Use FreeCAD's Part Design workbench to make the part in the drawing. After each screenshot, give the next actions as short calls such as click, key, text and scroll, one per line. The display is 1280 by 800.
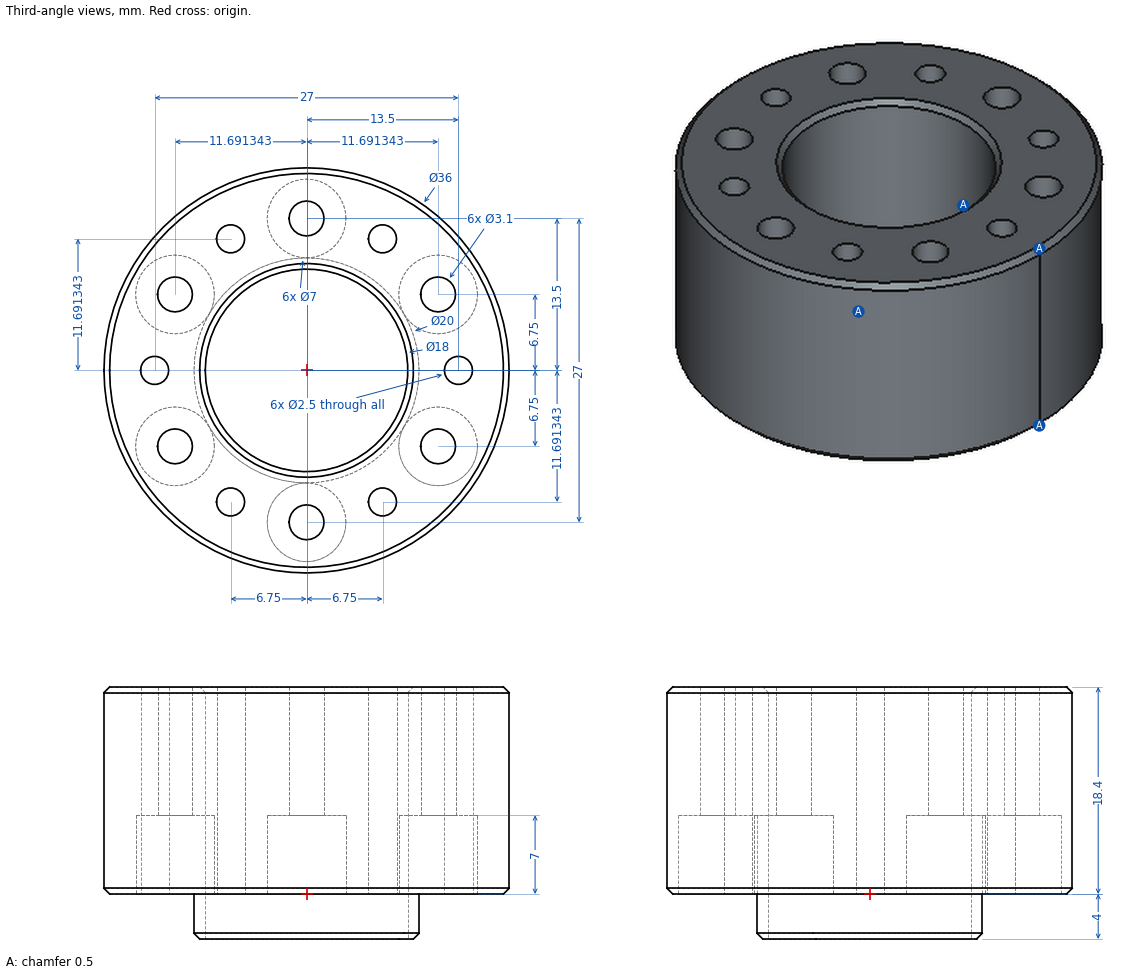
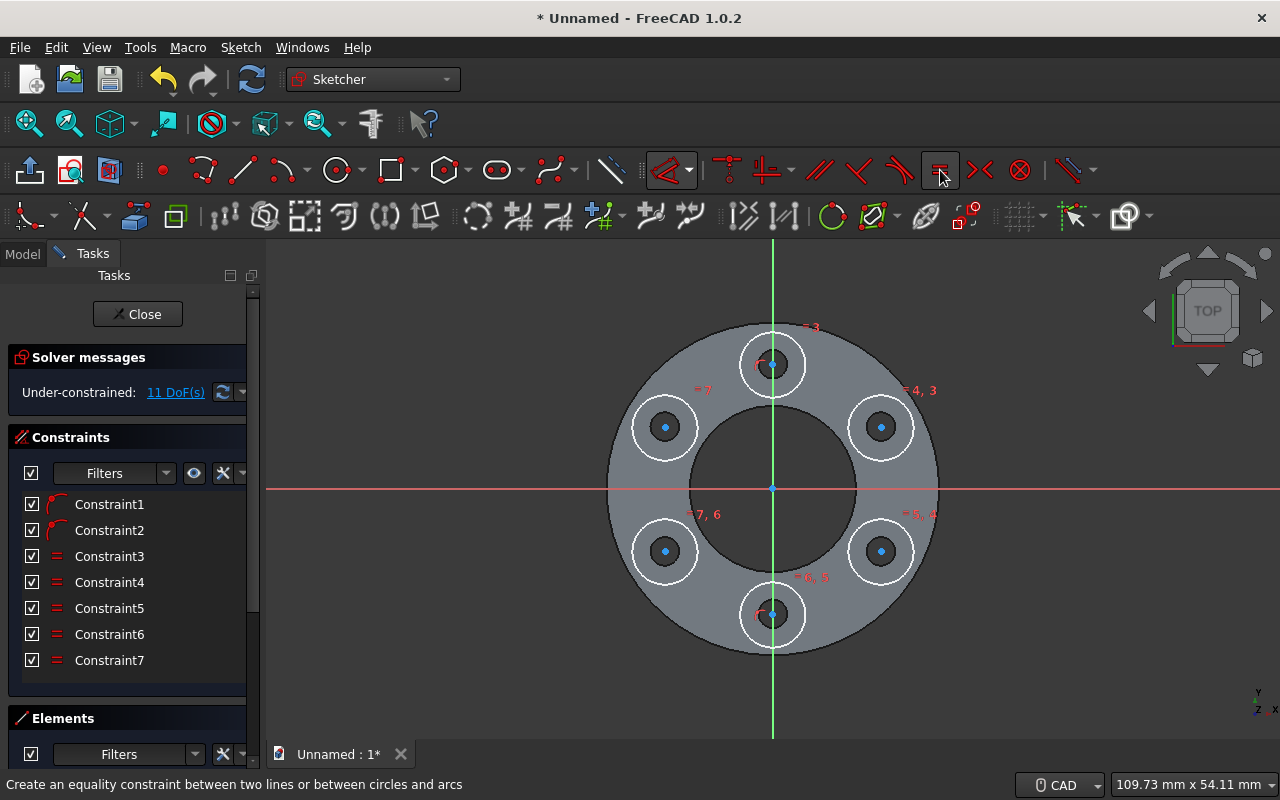
click(796, 342)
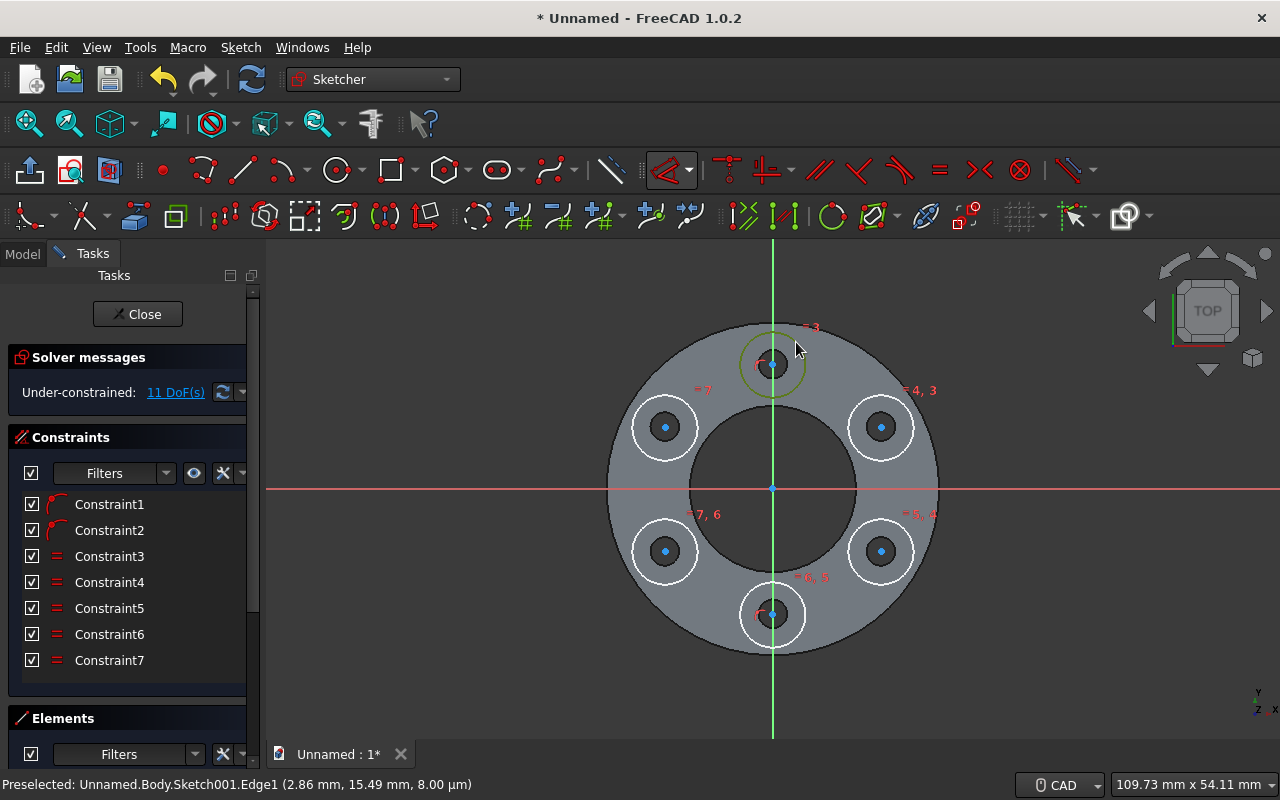
click(692, 170)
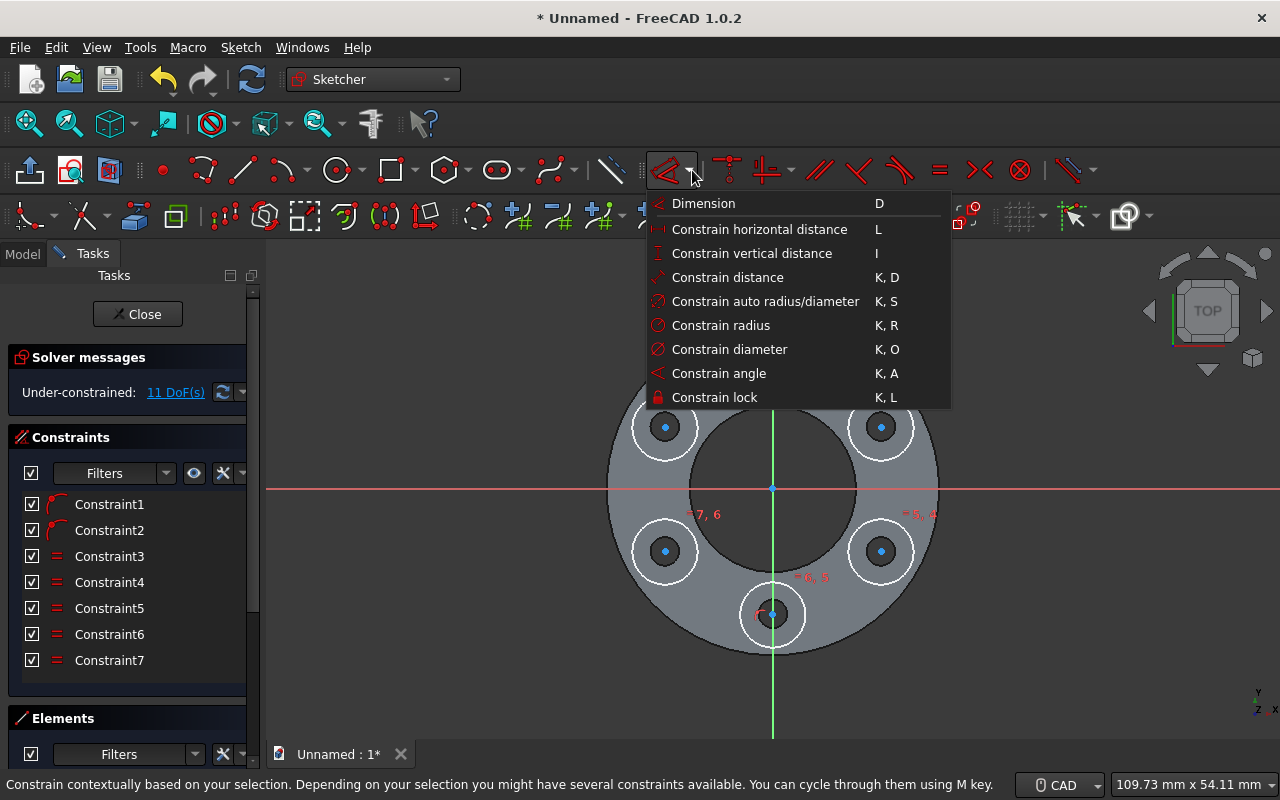
click(799, 349)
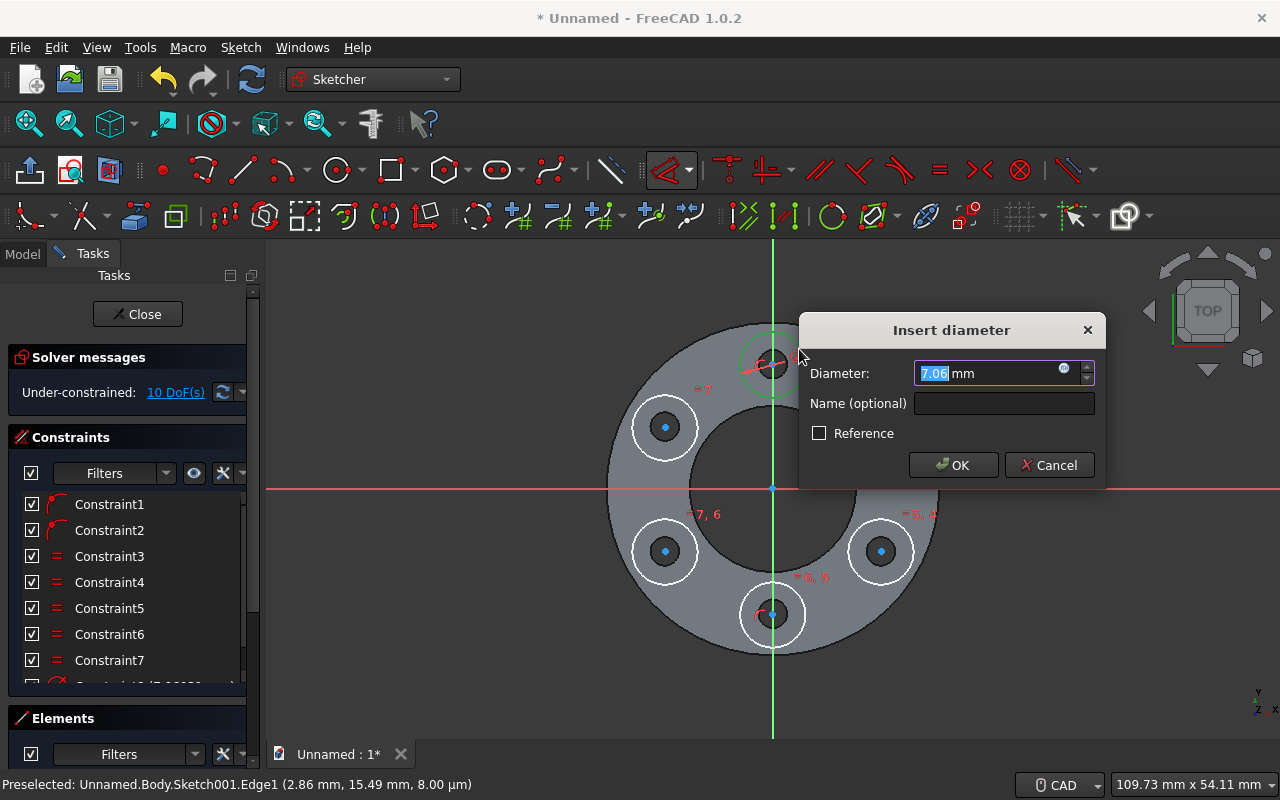
text(7)
key(Return)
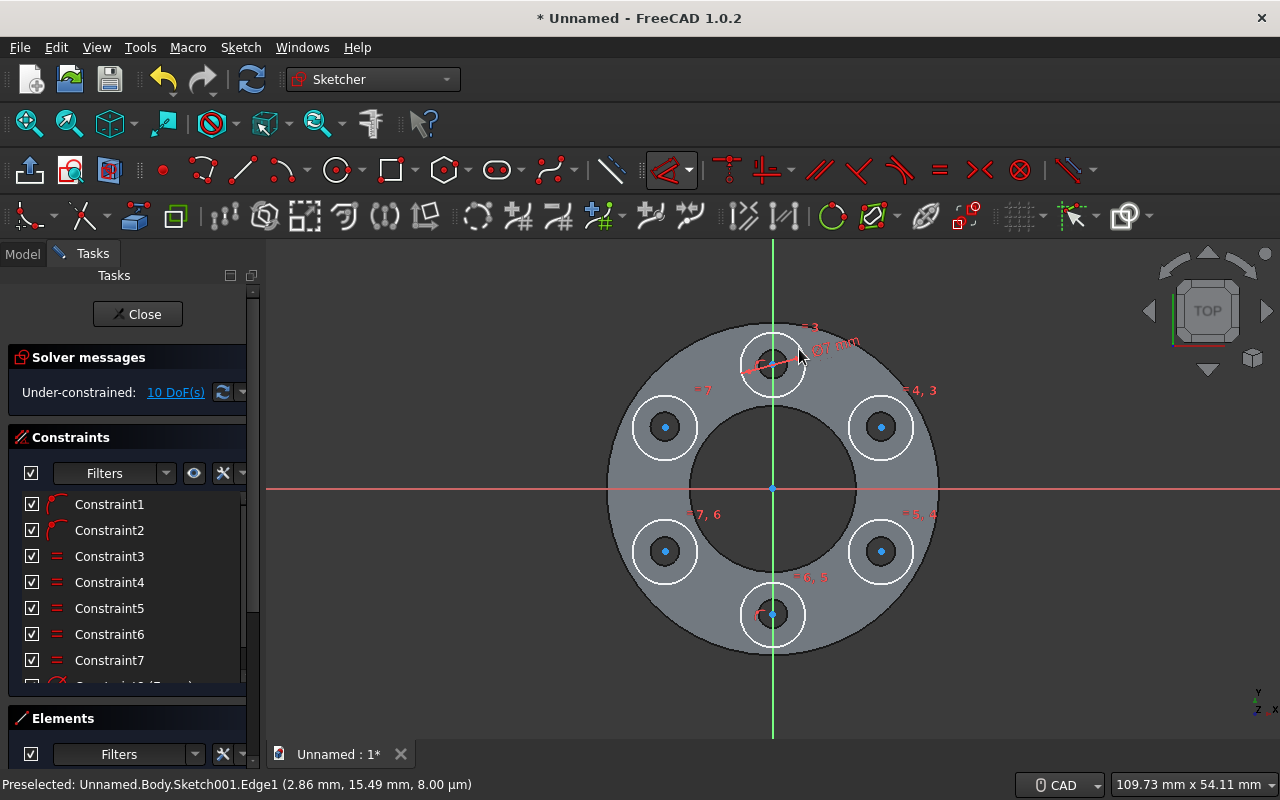
click(773, 365)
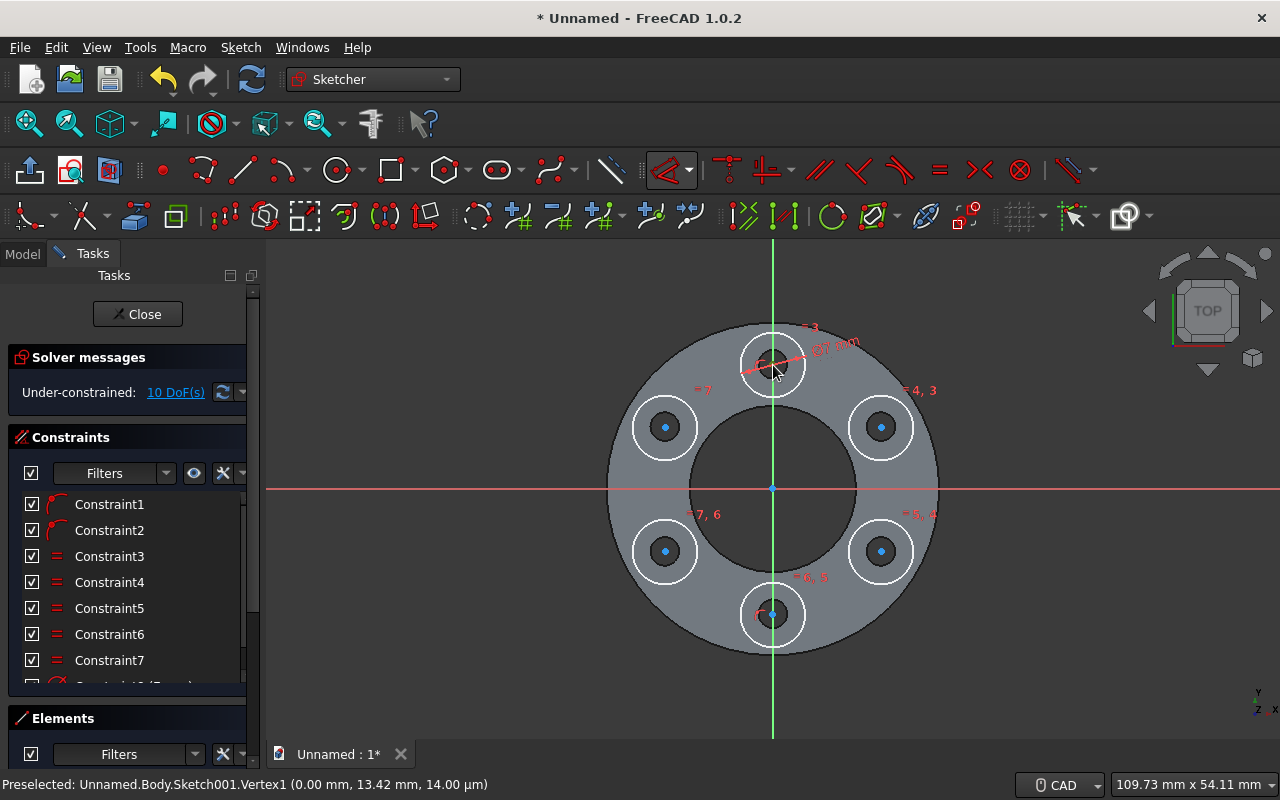
click(773, 615)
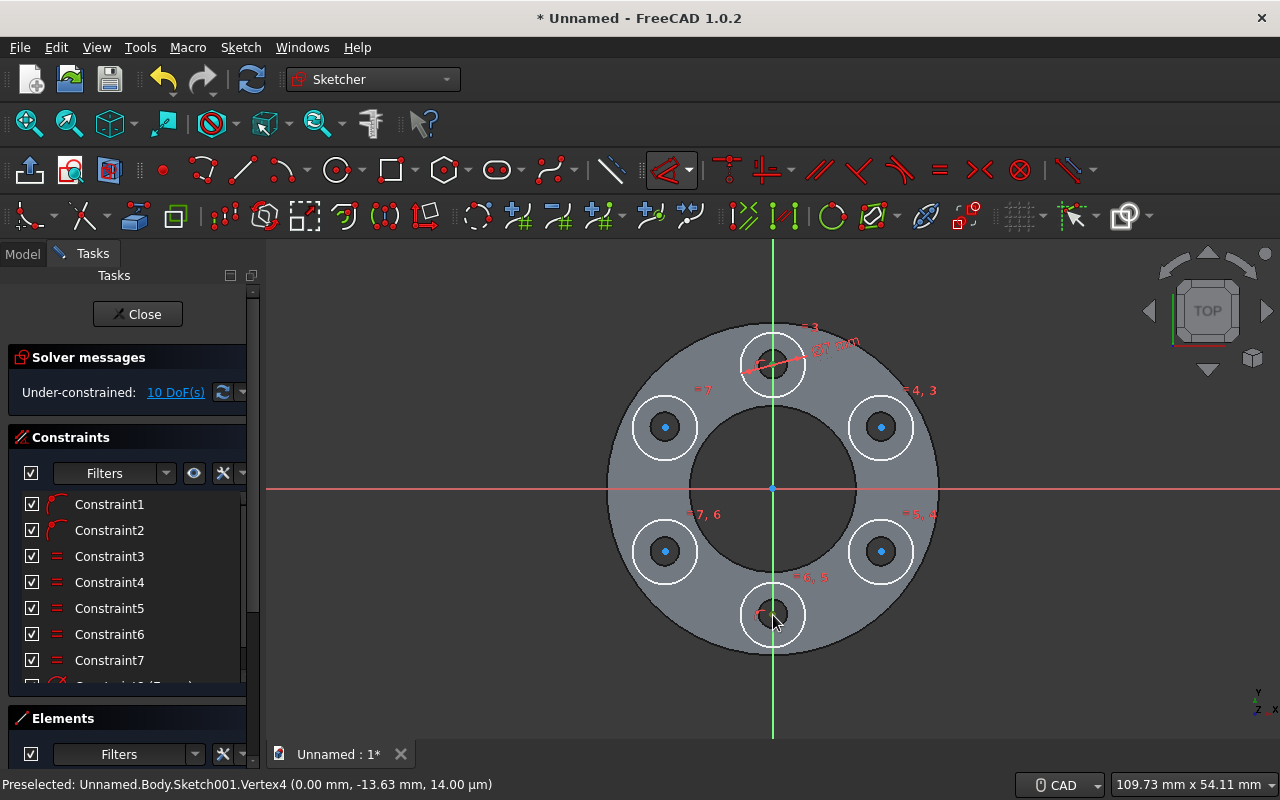
click(692, 170)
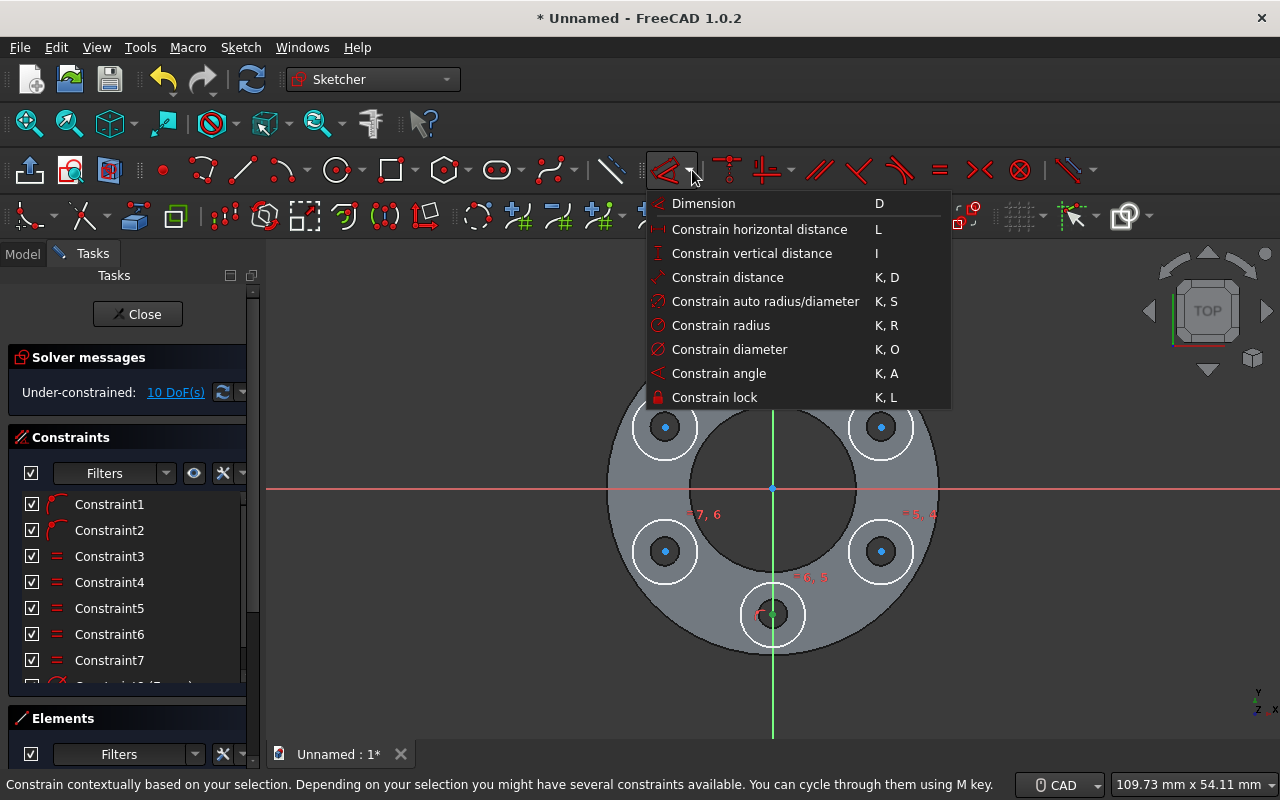
click(799, 253)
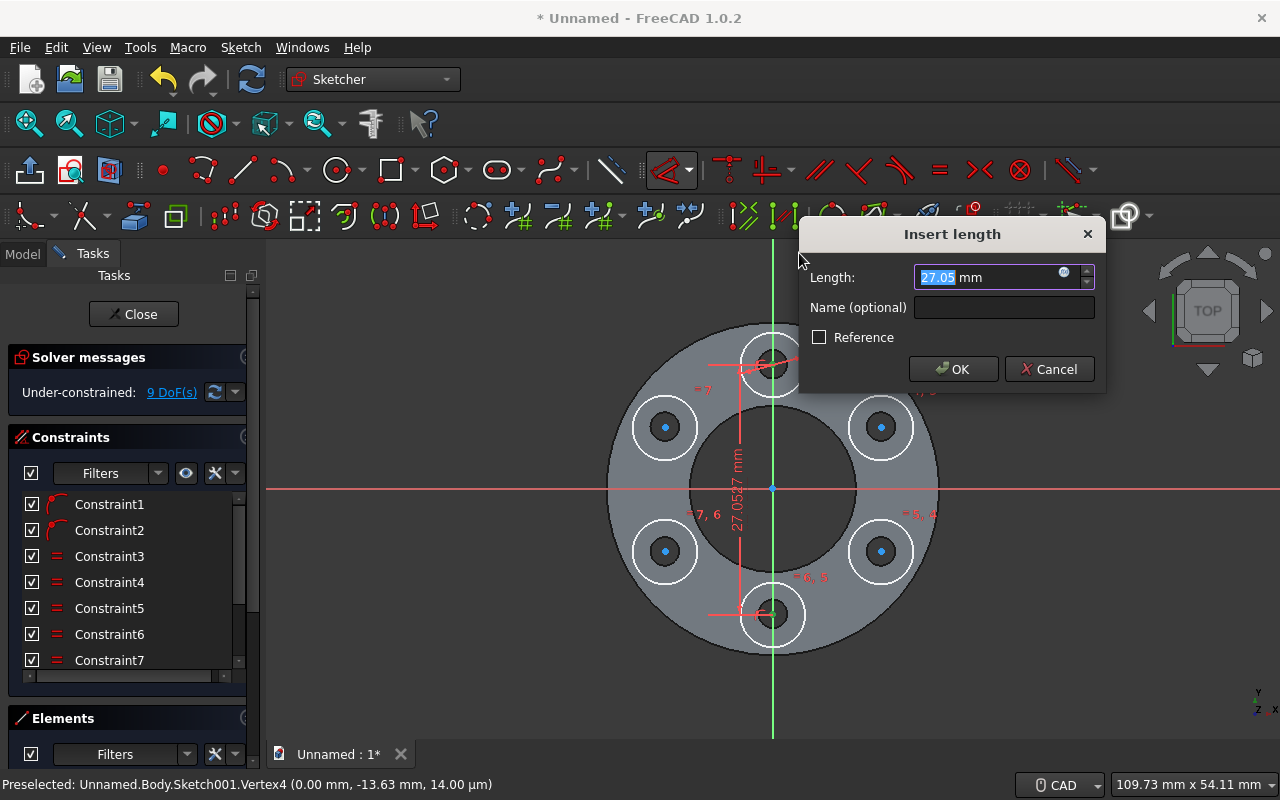
text(27)
key(Return)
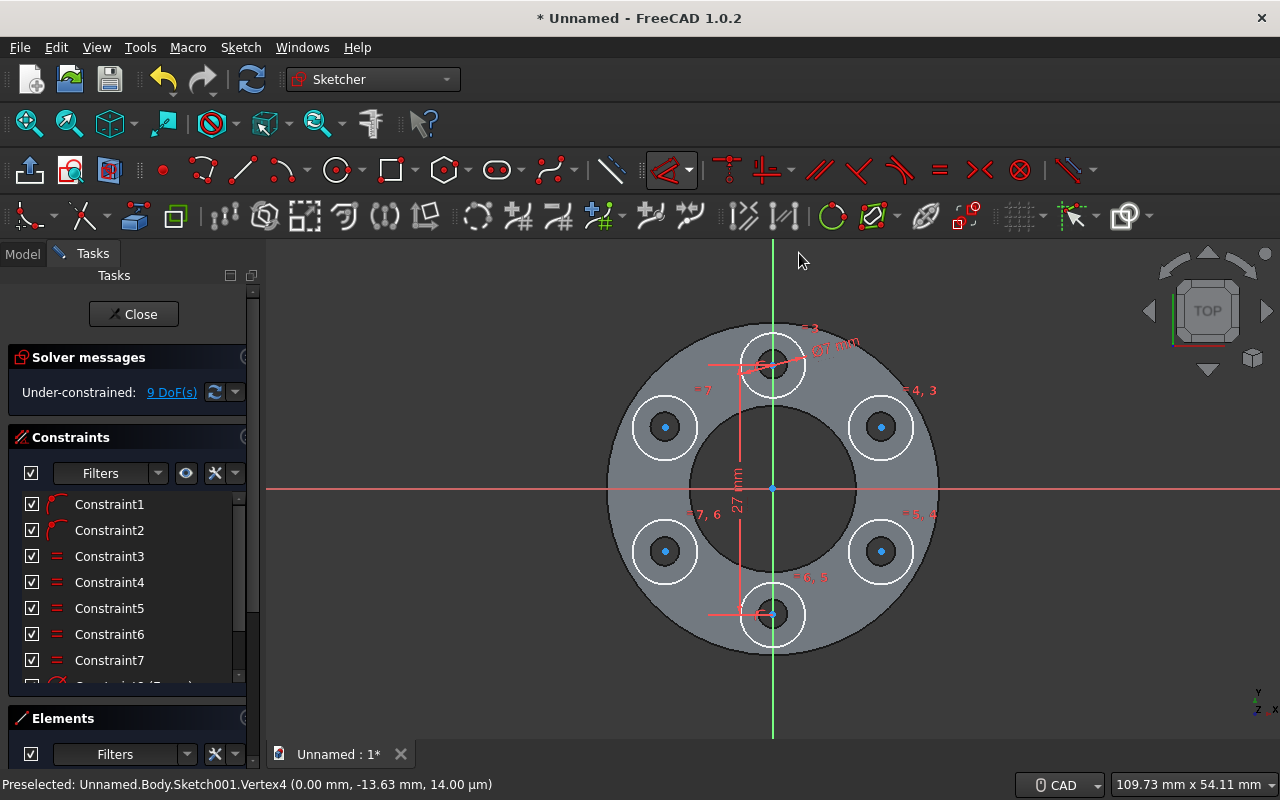
click(773, 365)